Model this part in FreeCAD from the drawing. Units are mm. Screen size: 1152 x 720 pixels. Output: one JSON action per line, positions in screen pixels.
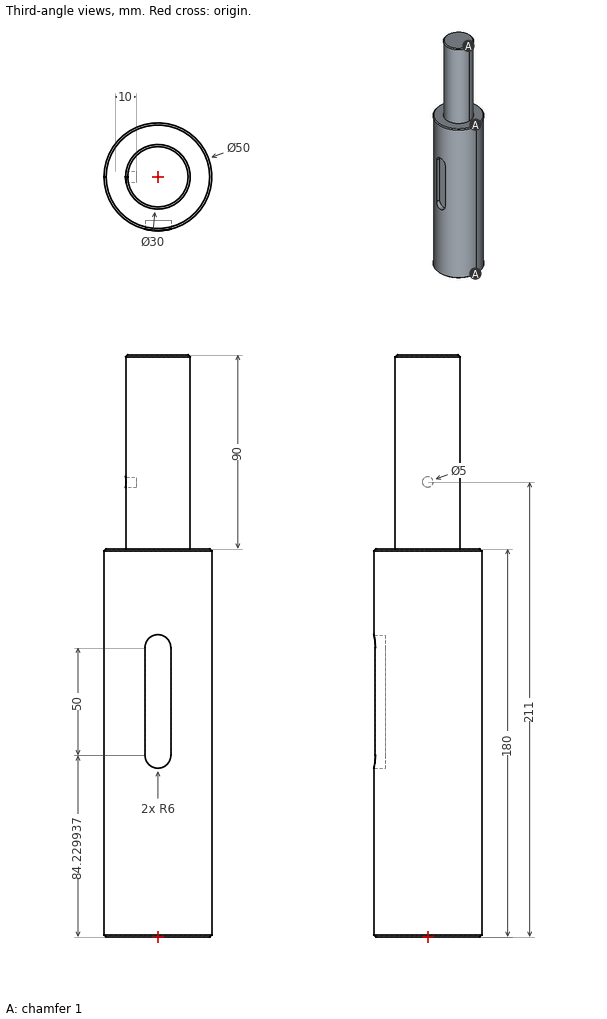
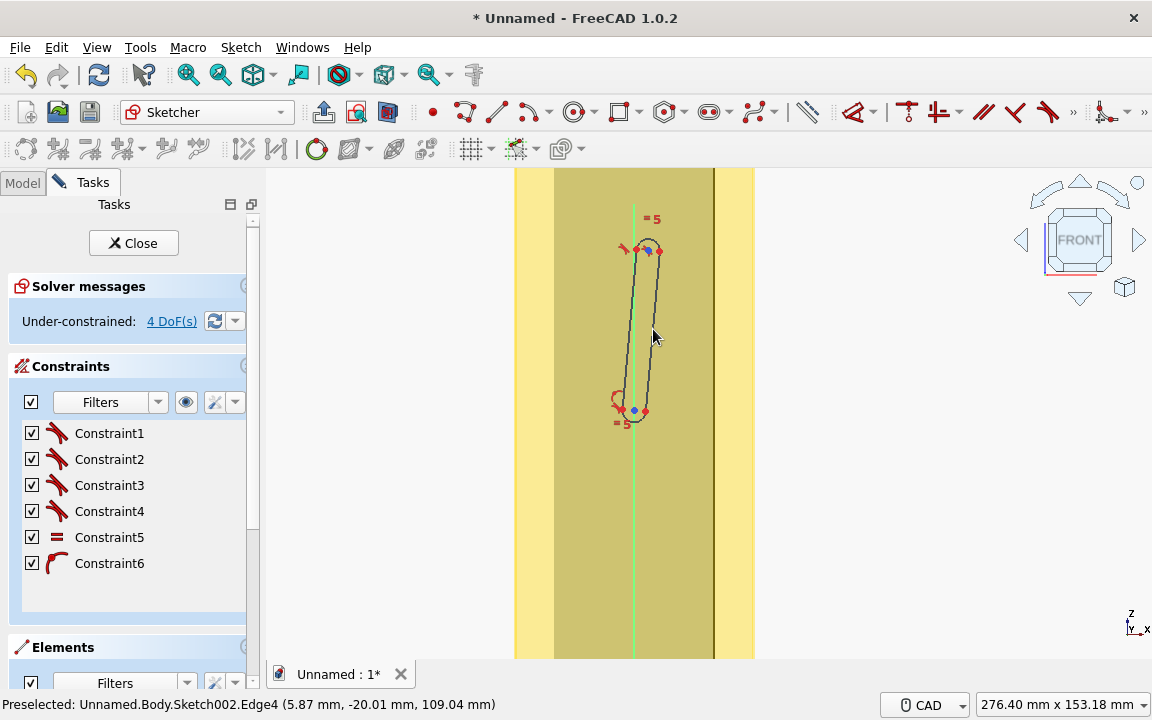
{"action": "left_click", "coordinate": [632, 298]}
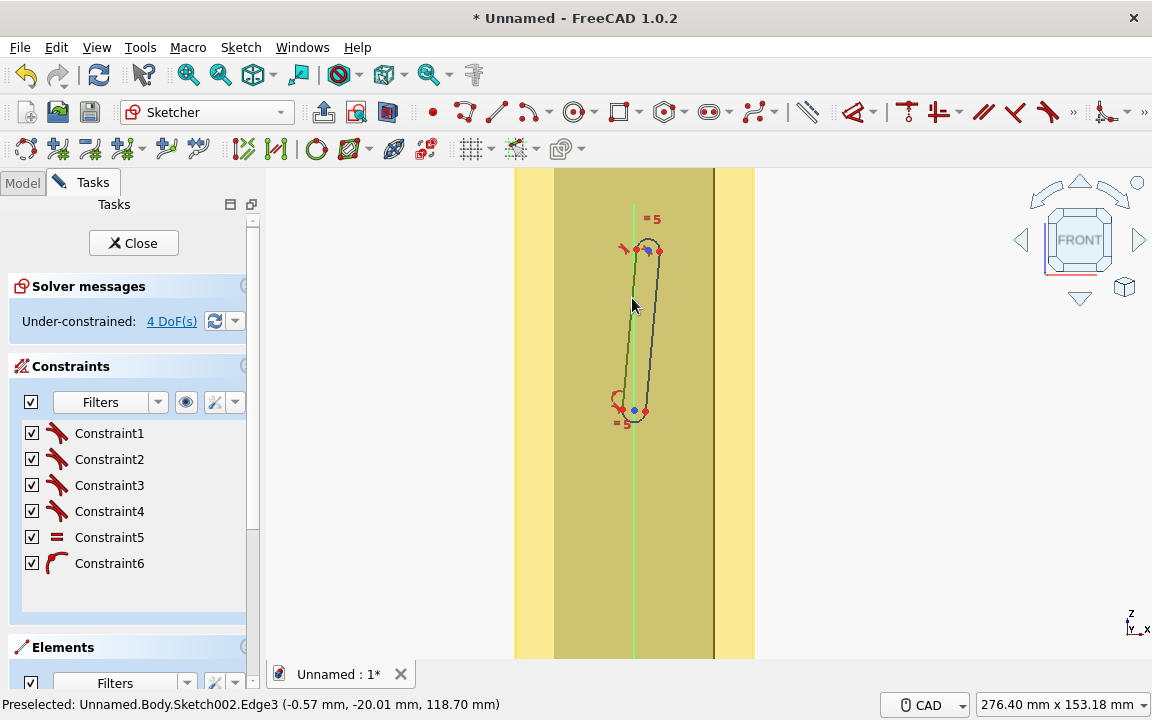
{"action": "key", "text": "v"}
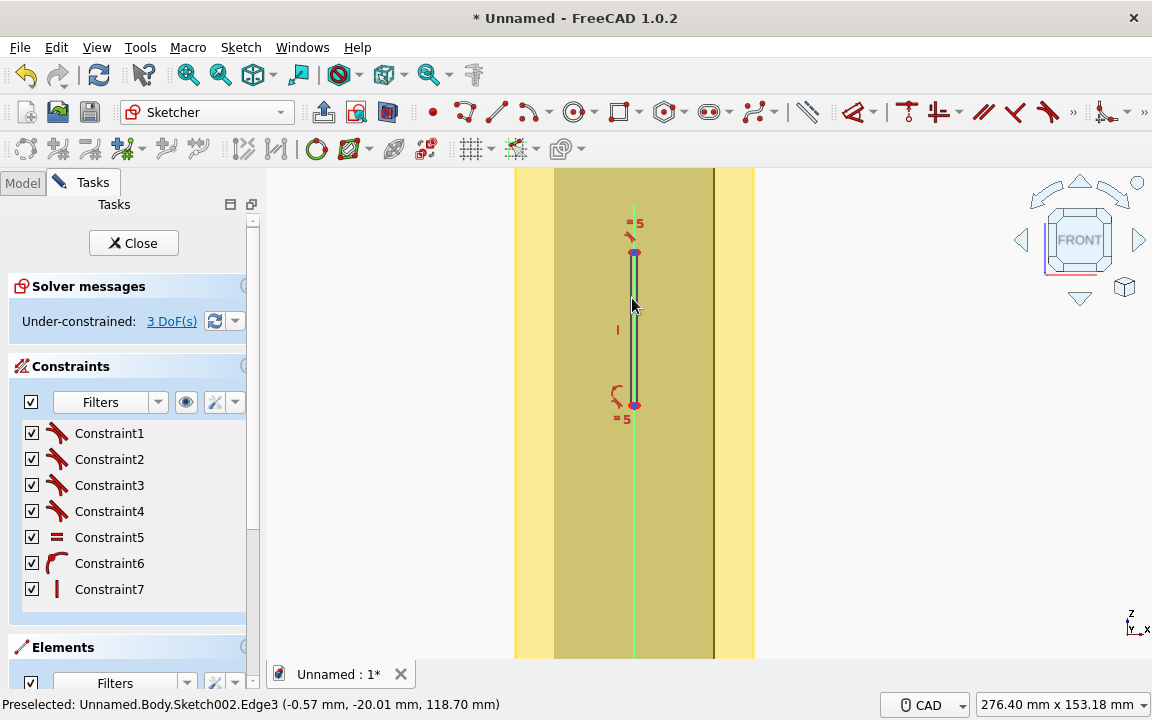
{"action": "left_click", "coordinate": [854, 112]}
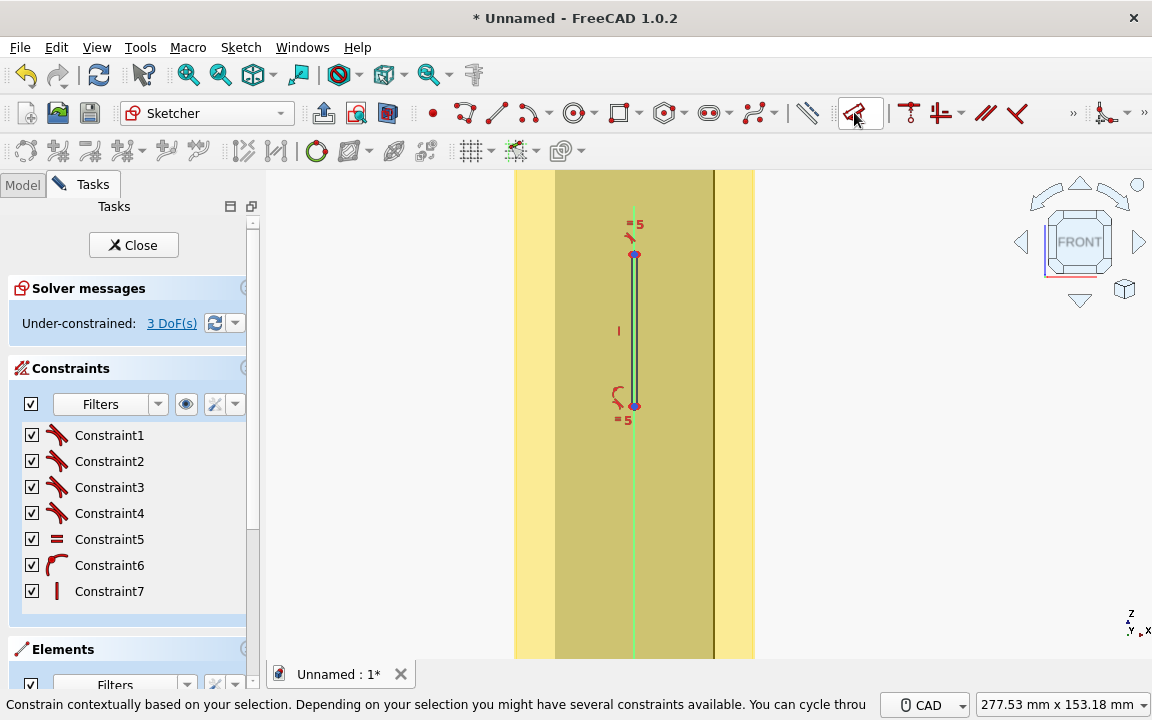
{"action": "scroll", "coordinate": [634, 410], "scroll_direction": "up", "scroll_amount": 8}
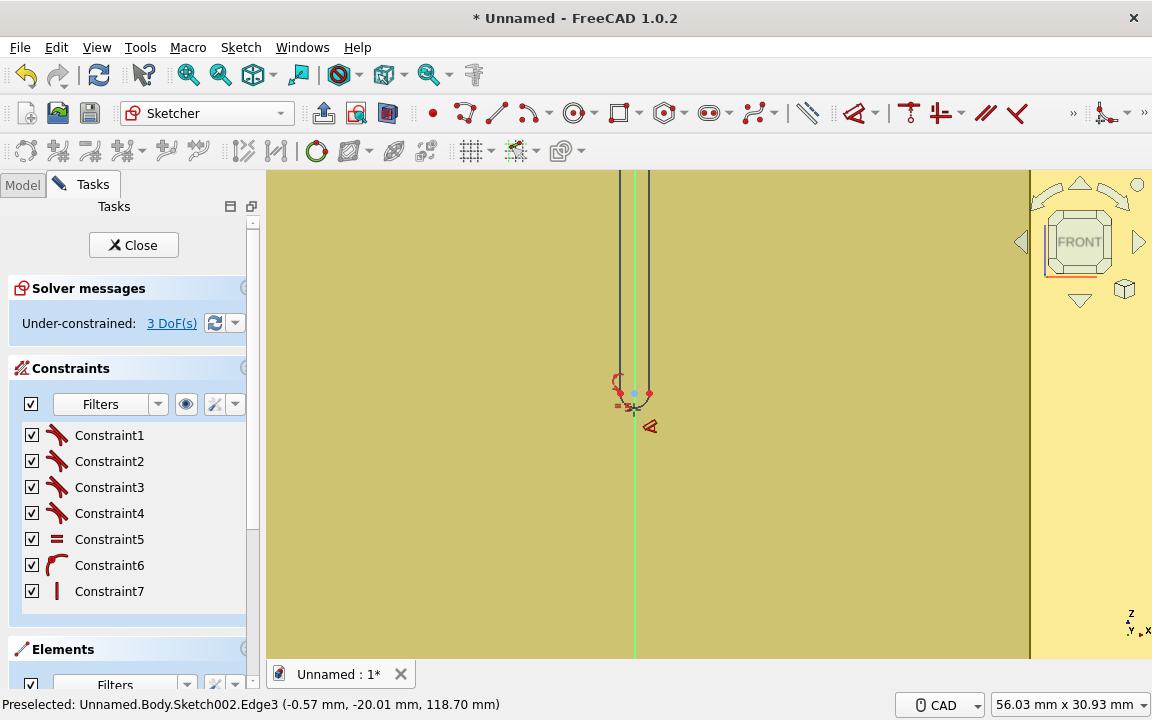
{"action": "left_click", "coordinate": [635, 408]}
{"action": "left_click", "coordinate": [613, 435]}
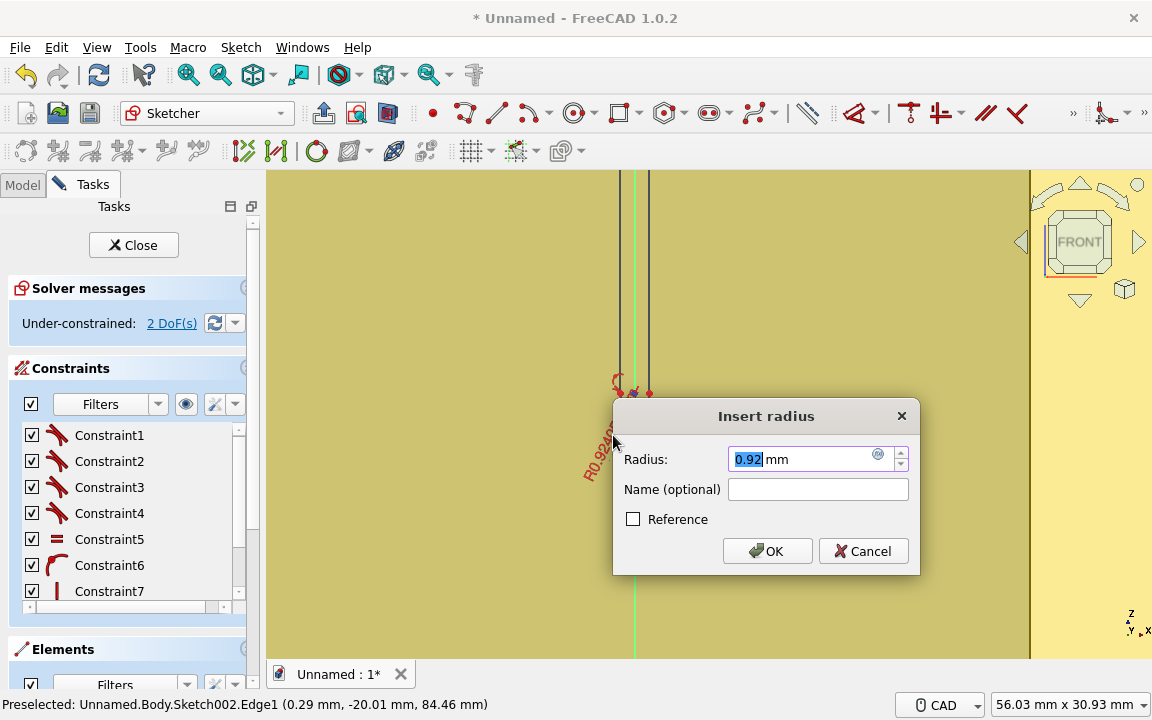
{"action": "type", "text": "6"}
{"action": "key", "text": "Return"}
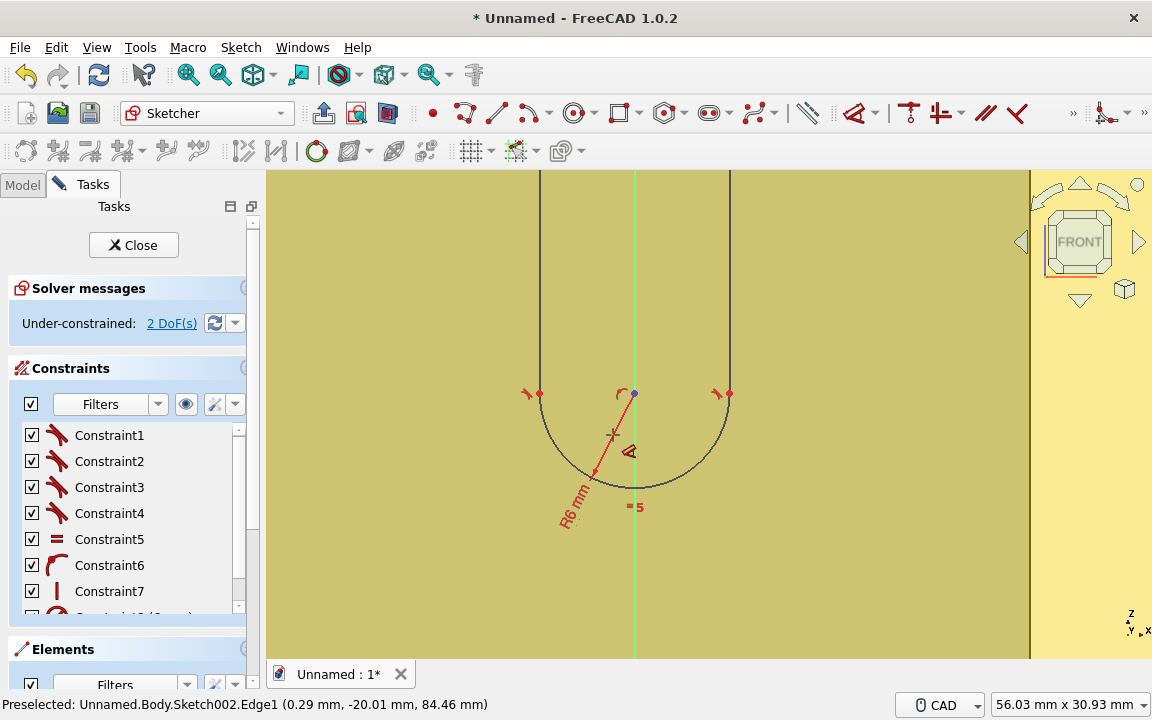
{"action": "scroll", "coordinate": [641, 380], "scroll_direction": "down", "scroll_amount": 10}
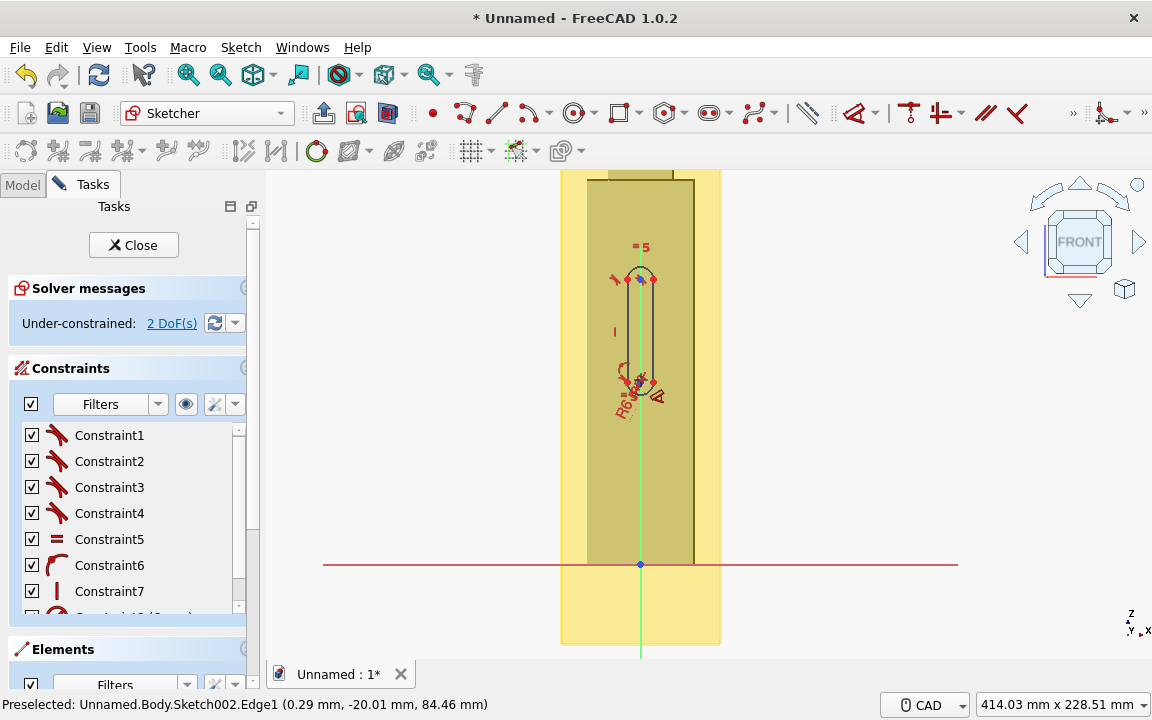
{"action": "left_click", "coordinate": [628, 362]}
{"action": "left_click", "coordinate": [594, 331]}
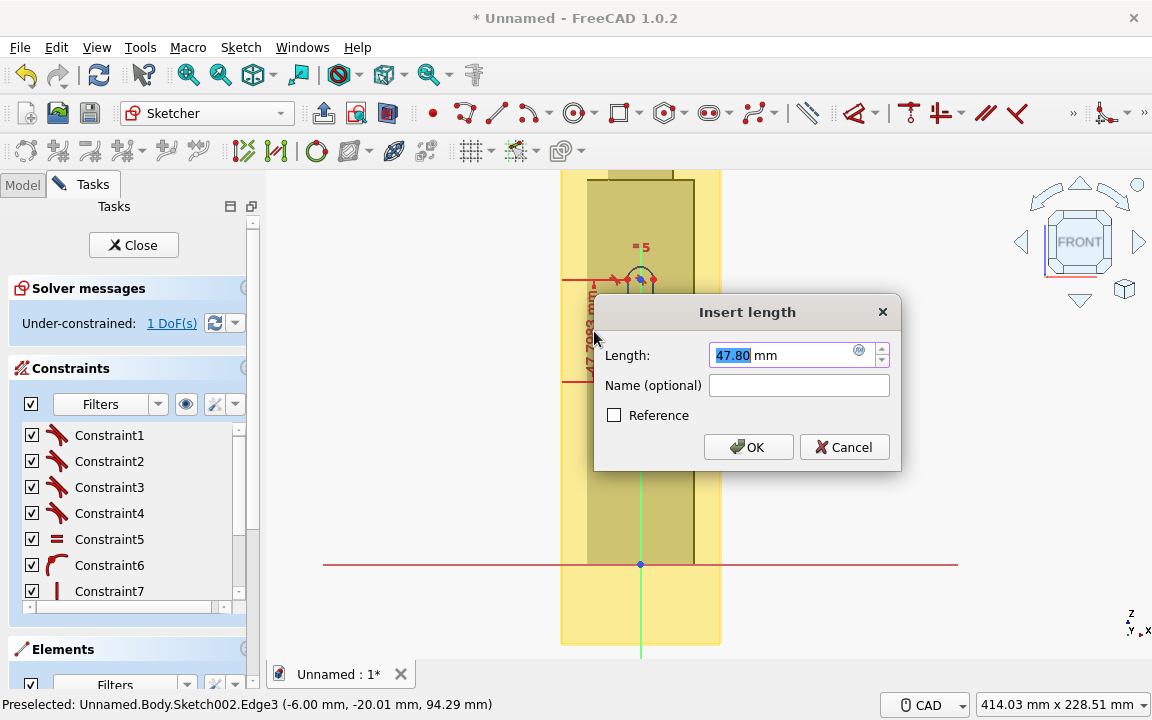
{"action": "type", "text": "50"}
{"action": "key", "text": "Return"}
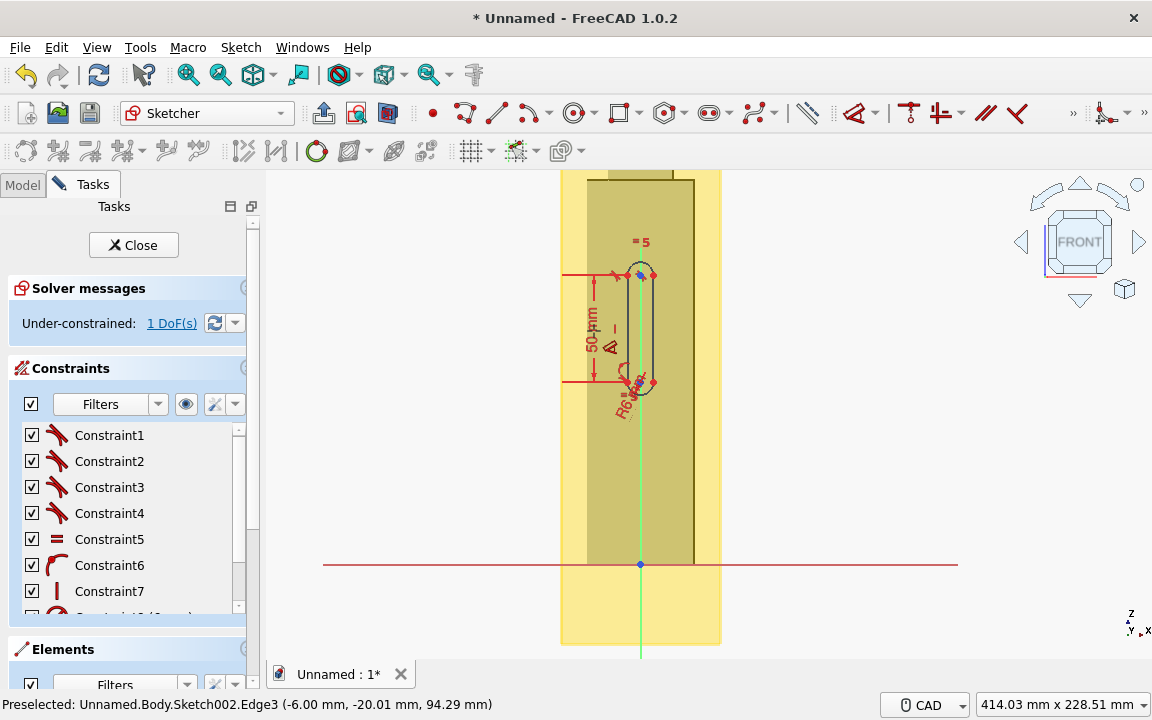
{"action": "left_click", "coordinate": [628, 382]}
{"action": "left_click", "coordinate": [594, 473]}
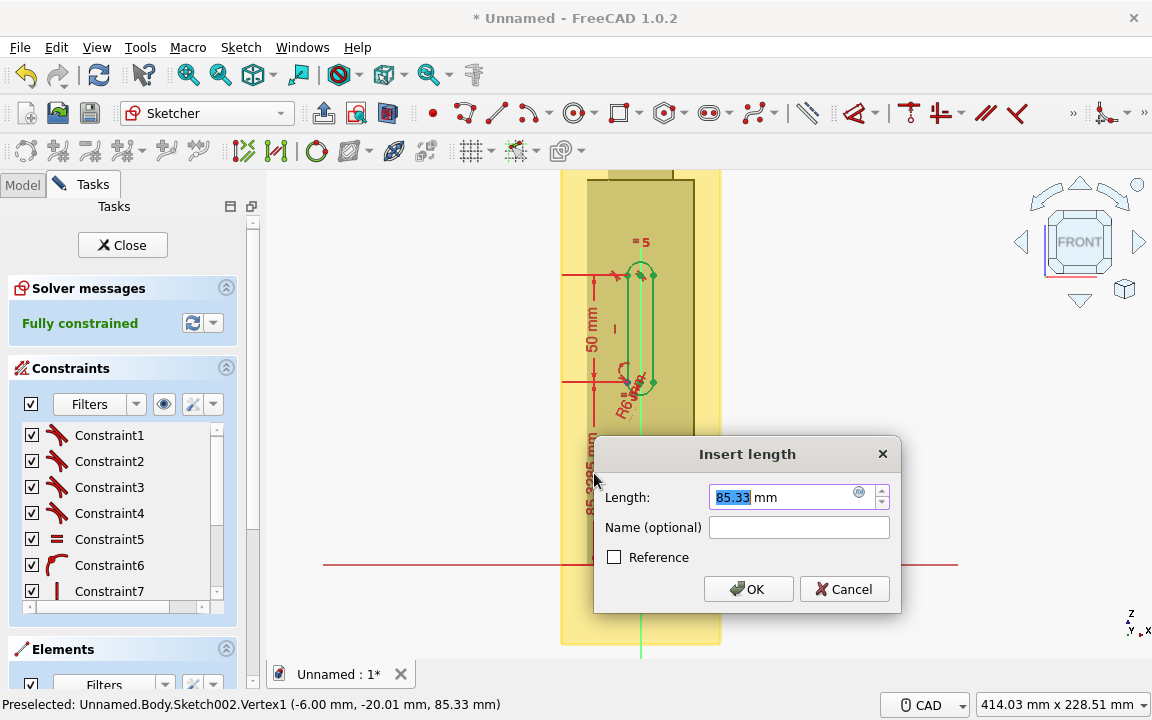
{"action": "type", "text": "84.229937"}
{"action": "key", "text": "Return"}
{"action": "key", "text": "Escape"}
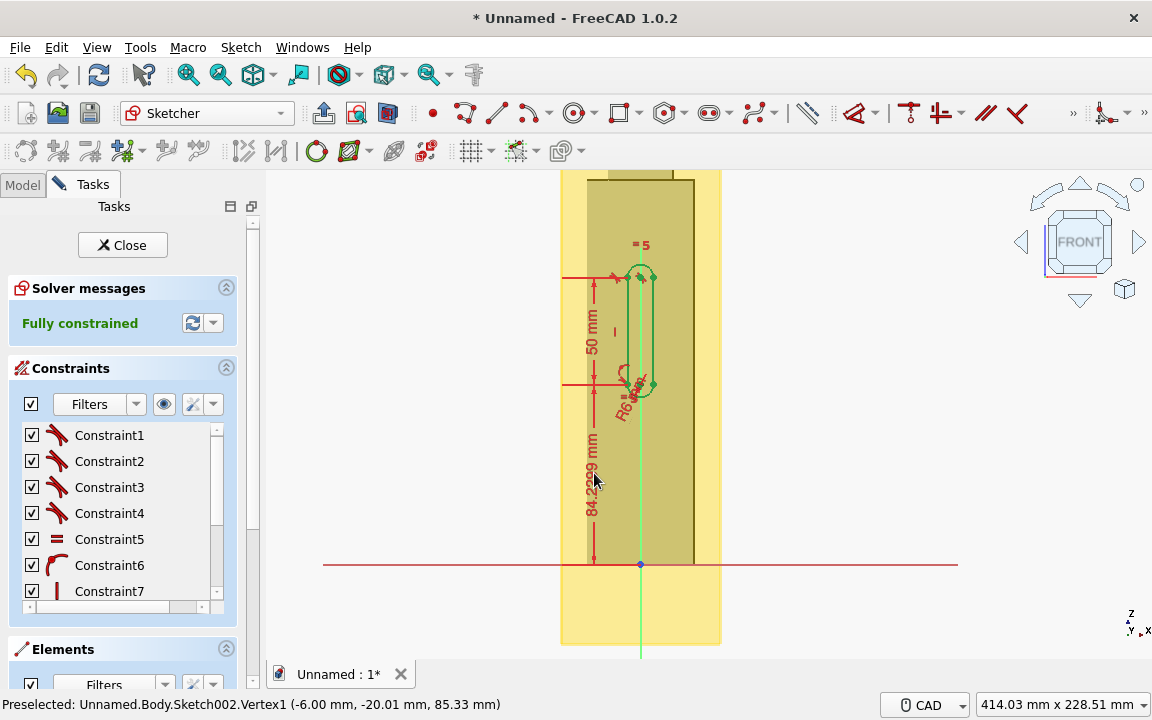
{"action": "left_click", "coordinate": [123, 245]}